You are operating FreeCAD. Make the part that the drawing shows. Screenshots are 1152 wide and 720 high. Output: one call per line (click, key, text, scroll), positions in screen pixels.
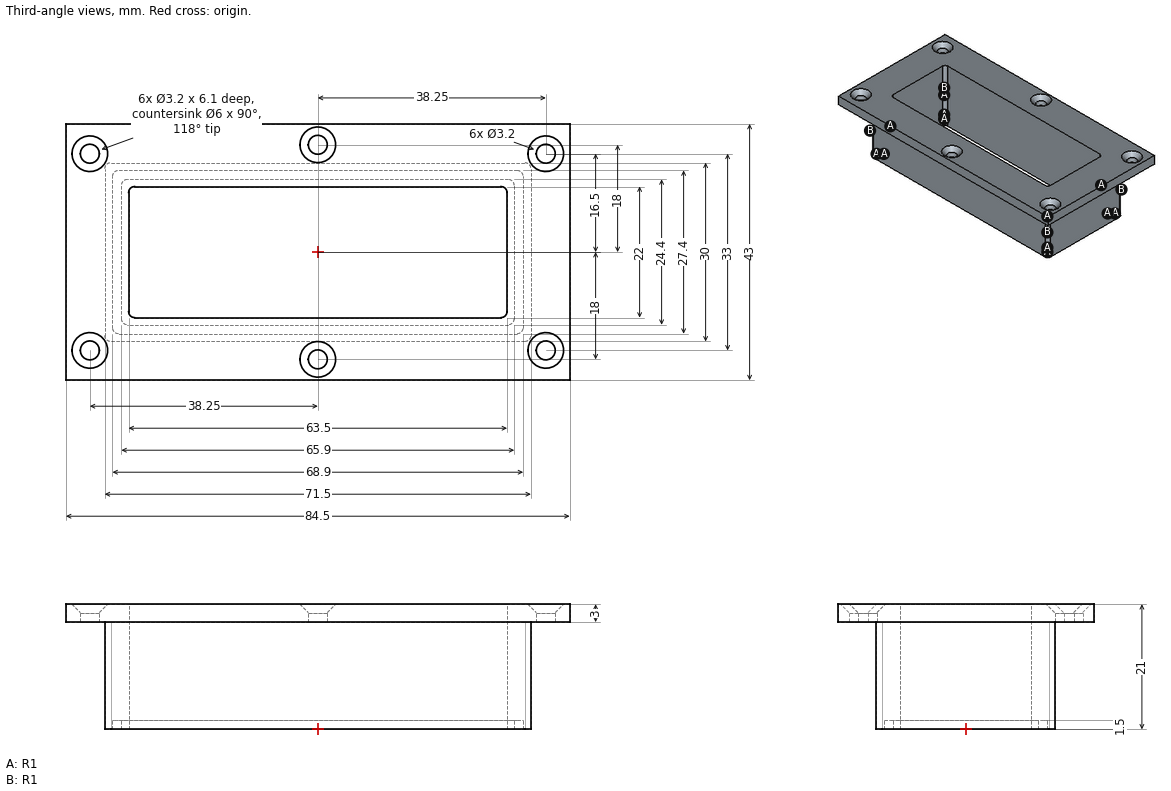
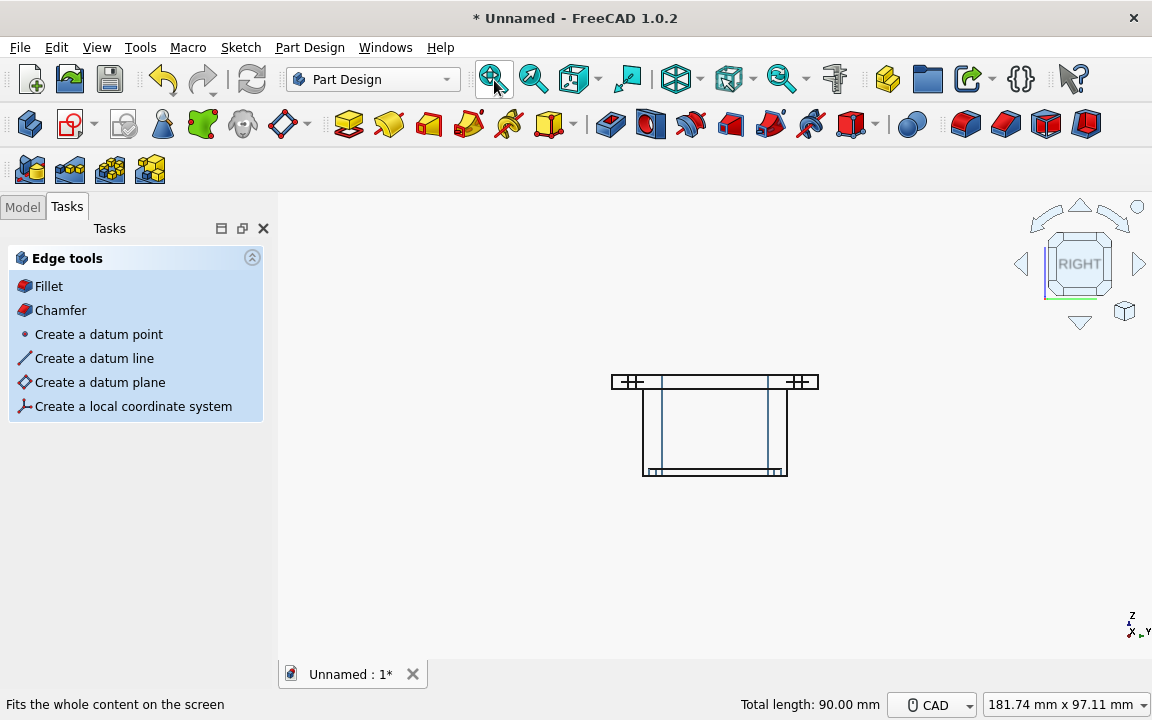
key(5)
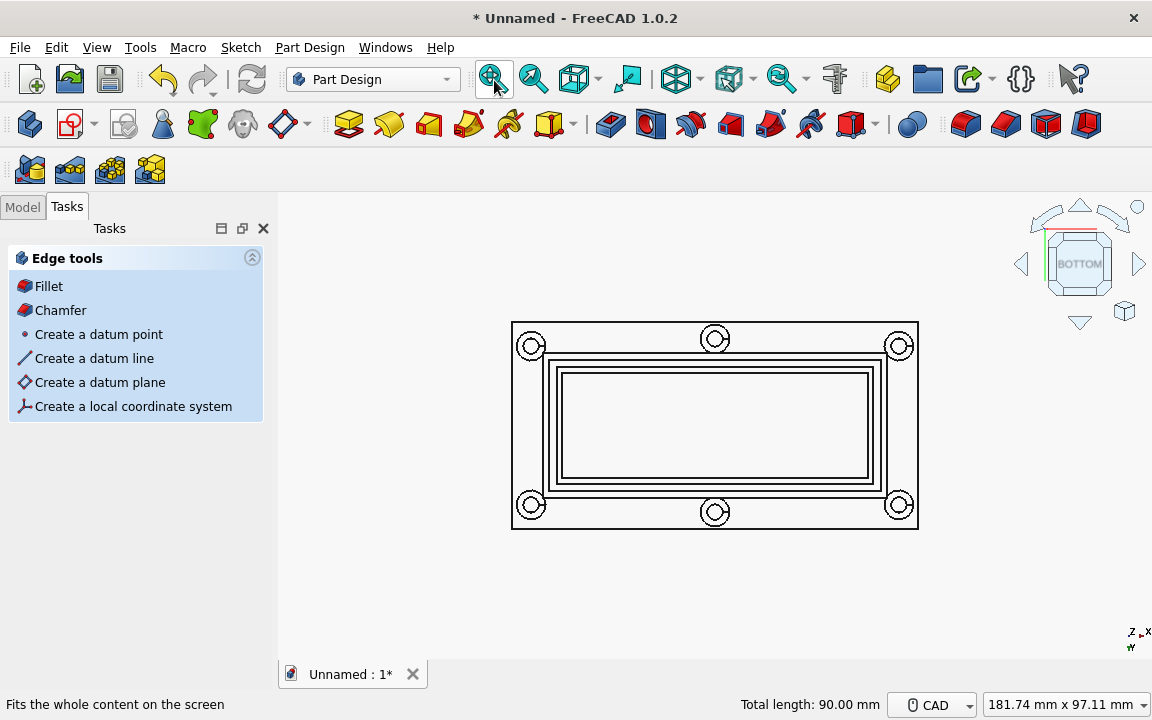
scroll(549, 490, up, 9)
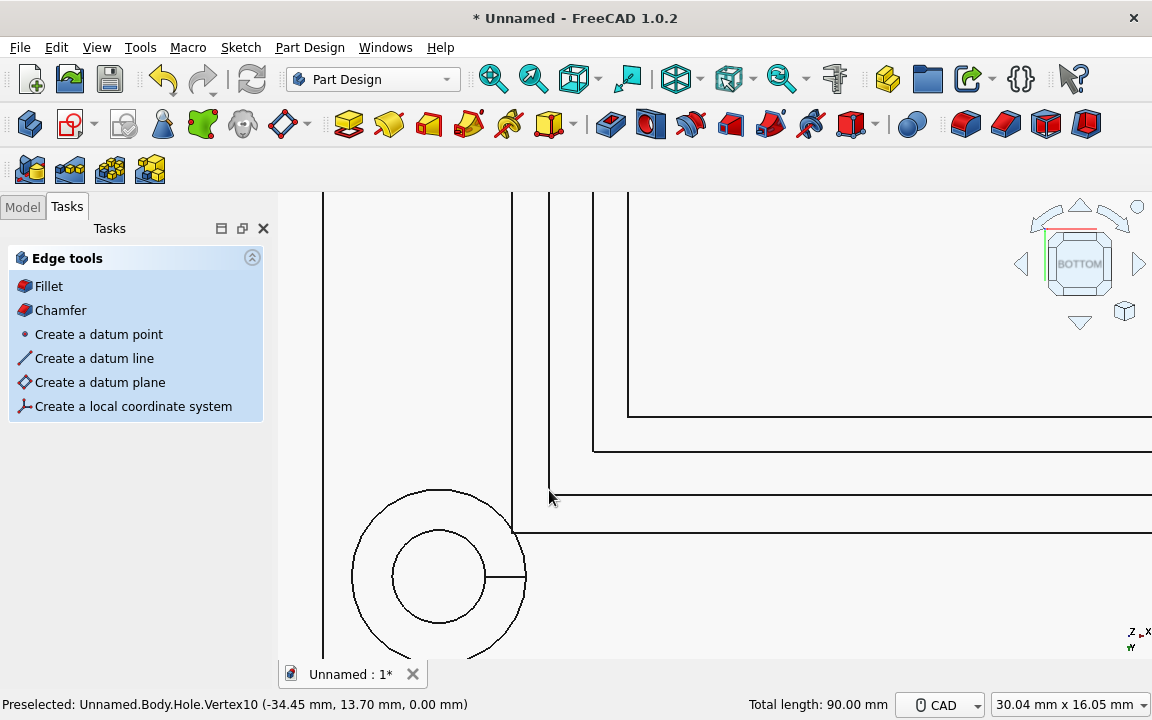
click(494, 80)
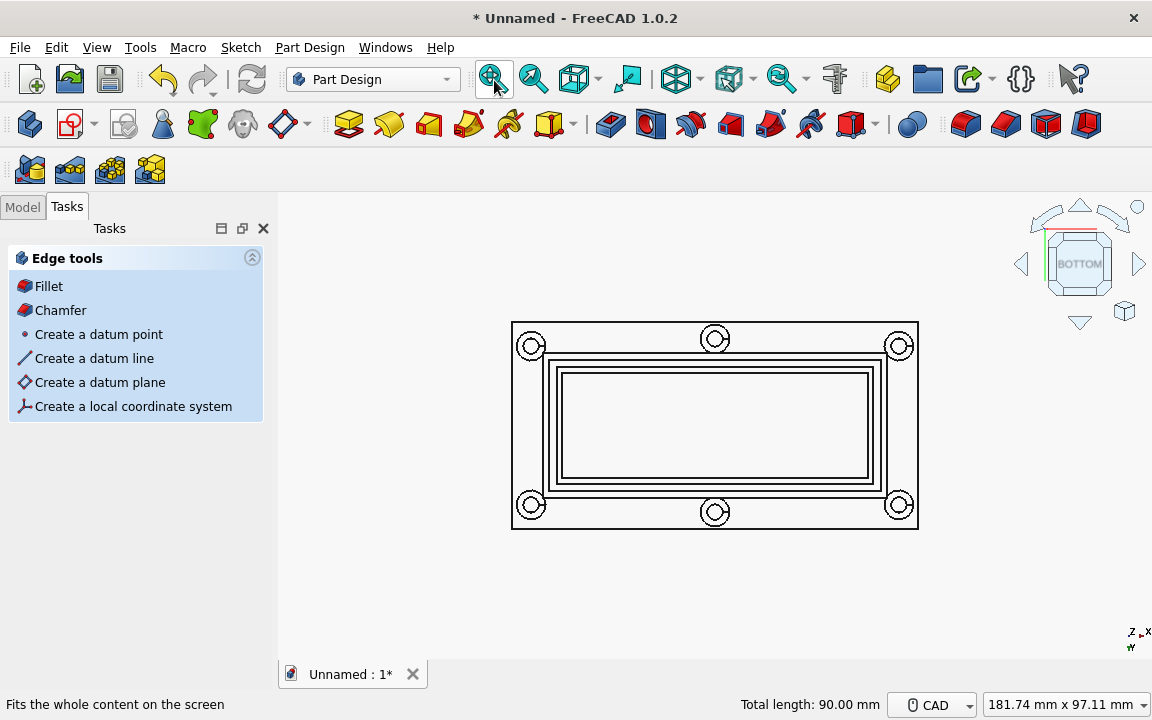
key(4)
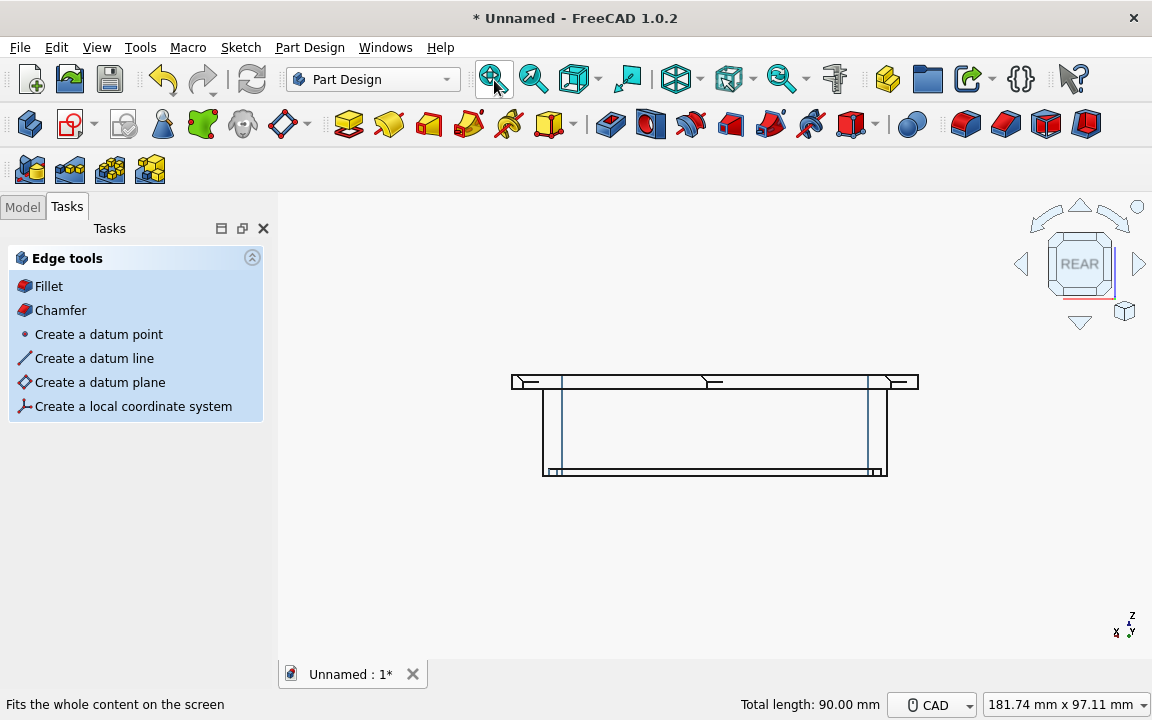
scroll(881, 471, up, 9)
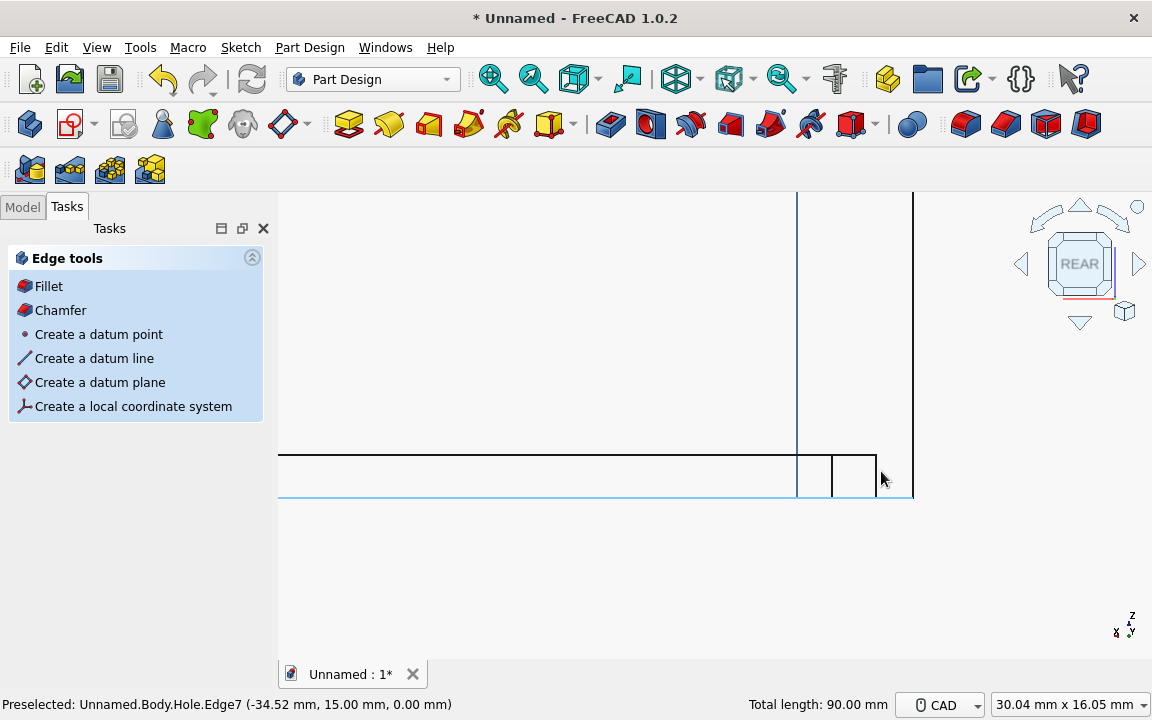
click(876, 475, ctrl)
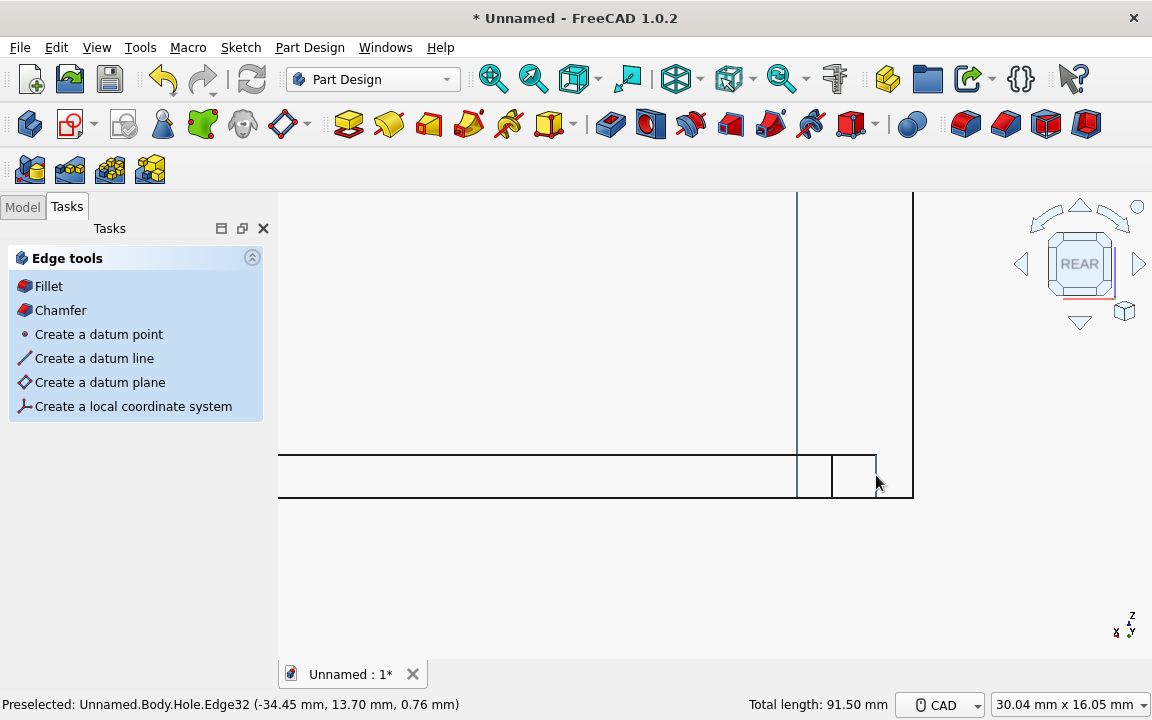
click(832, 475, ctrl)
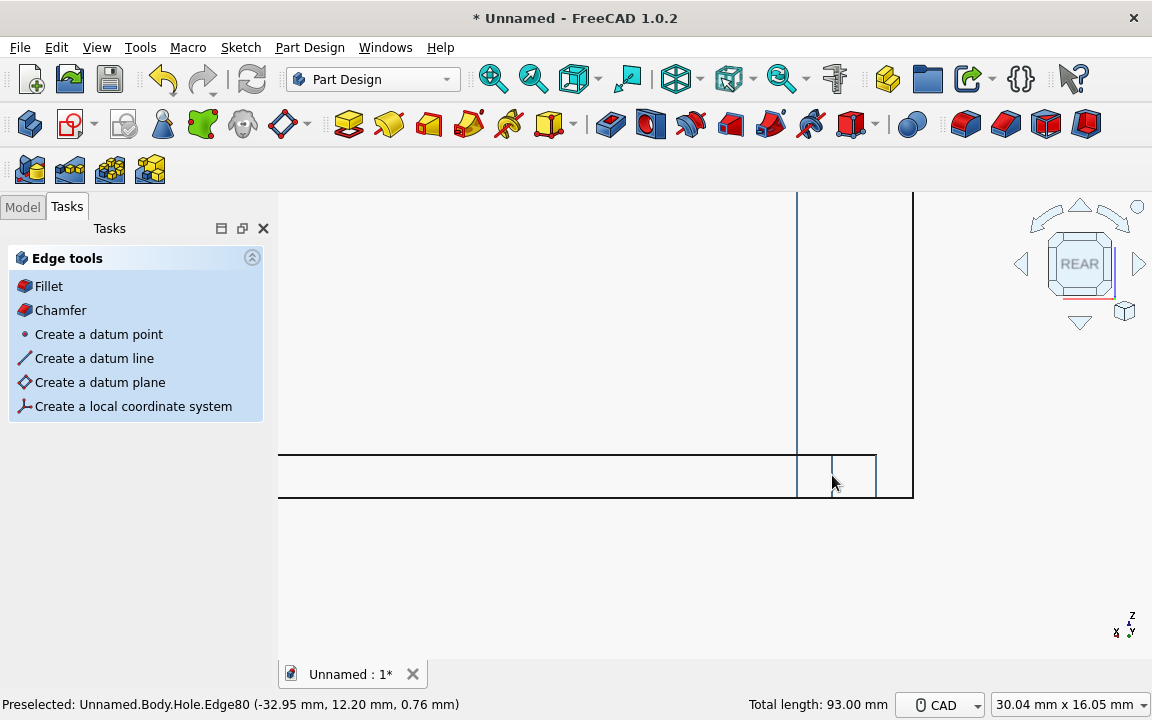
key(v)
key(f)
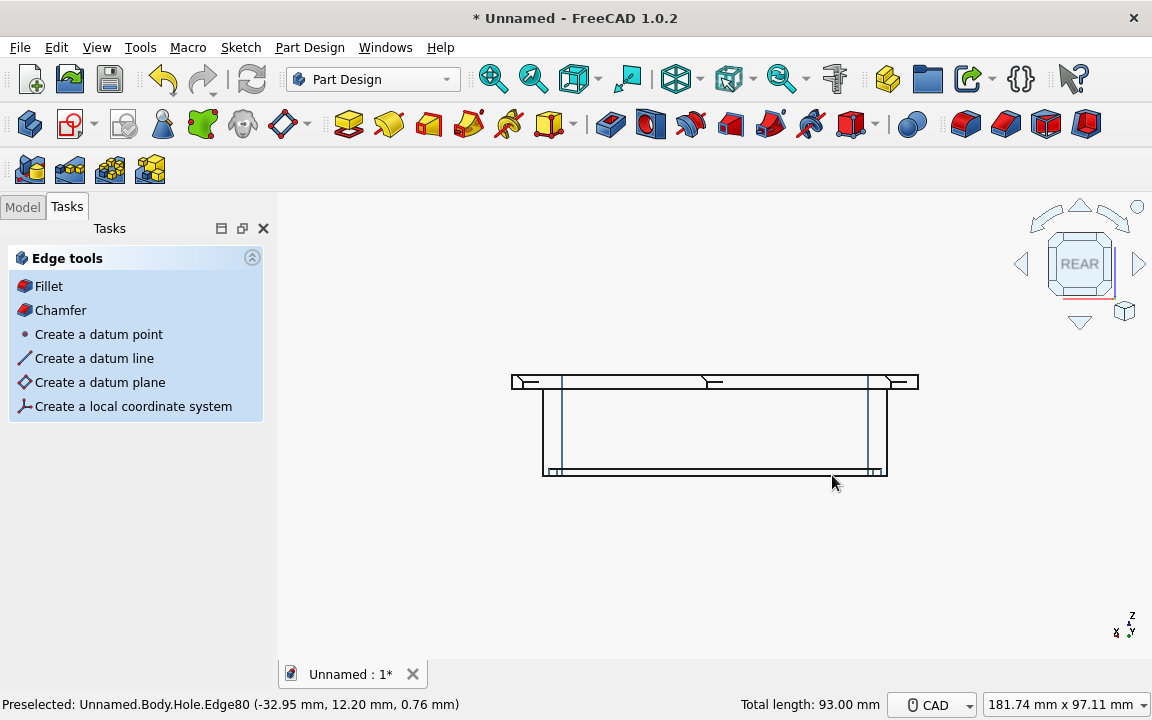
key(6)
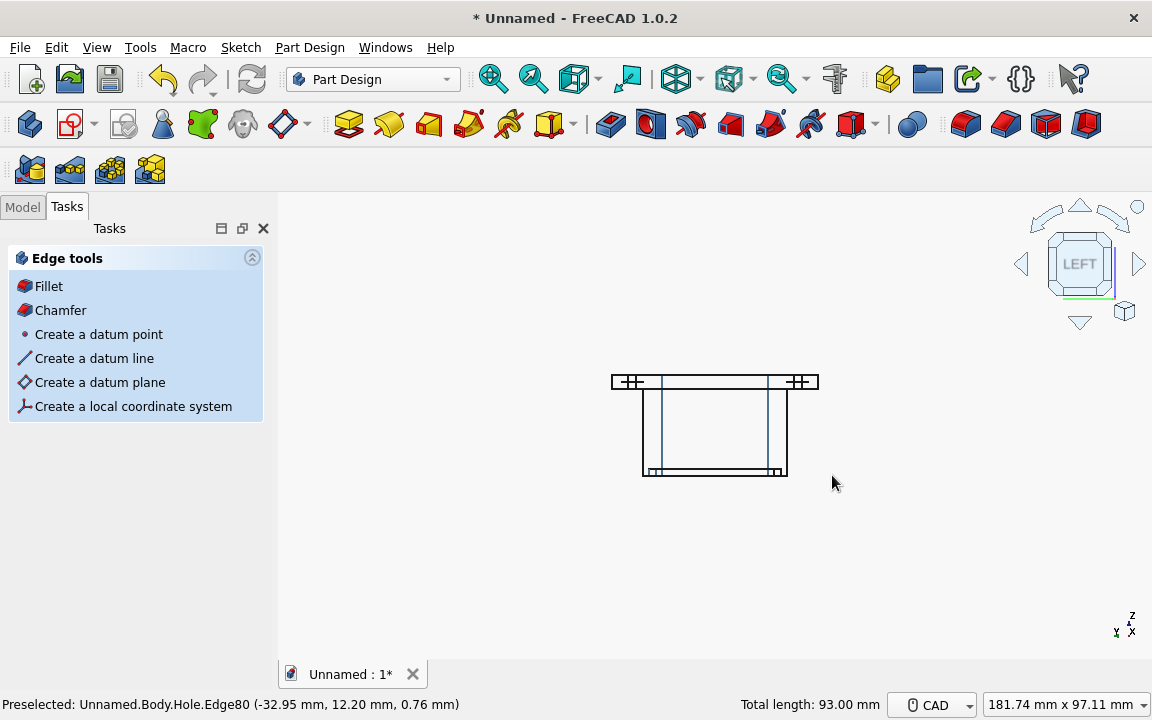
click(494, 80)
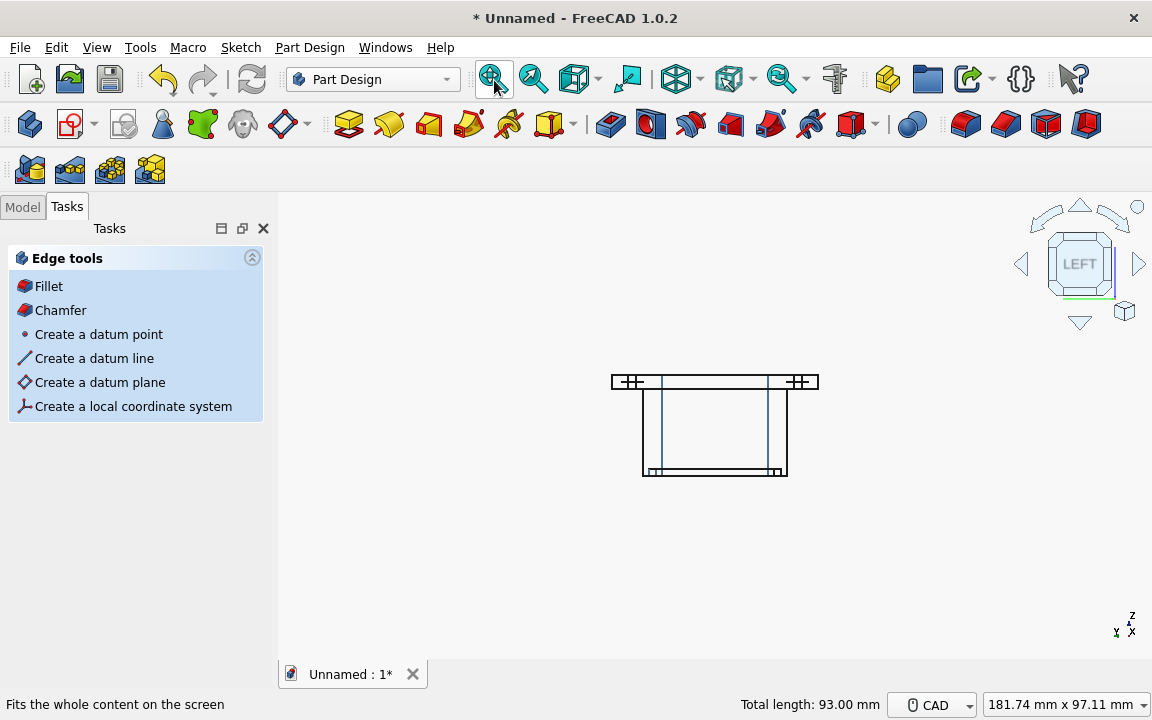
scroll(781, 471, up, 9)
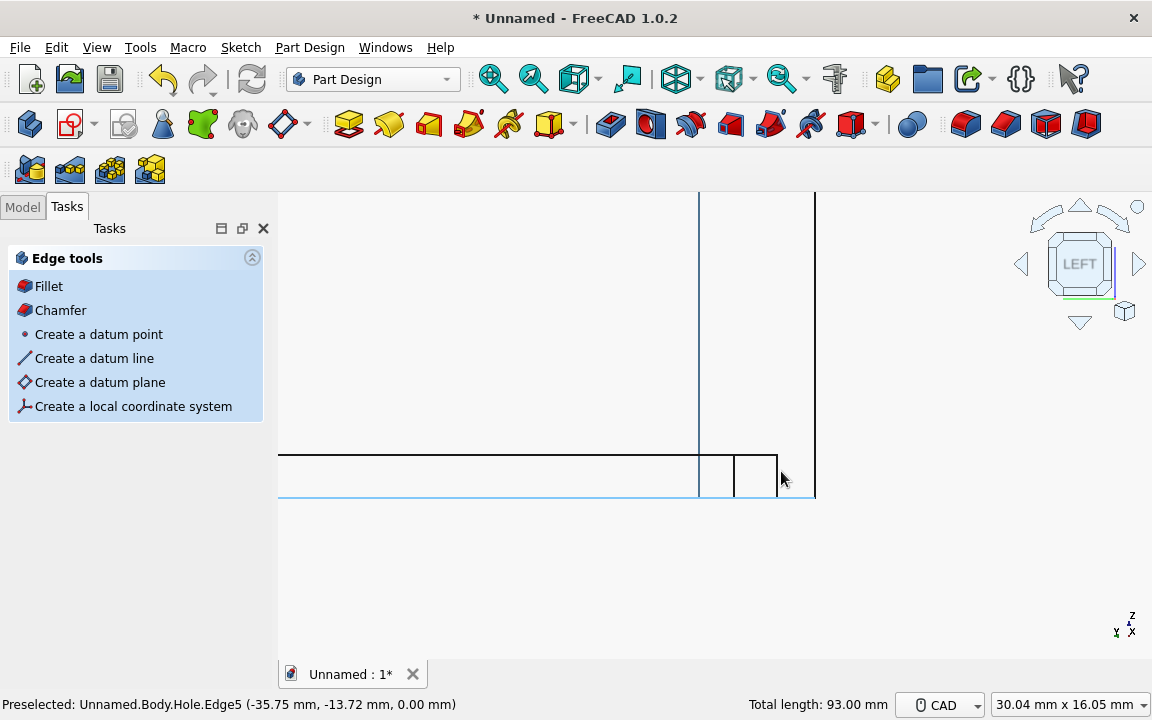
click(777, 475, ctrl)